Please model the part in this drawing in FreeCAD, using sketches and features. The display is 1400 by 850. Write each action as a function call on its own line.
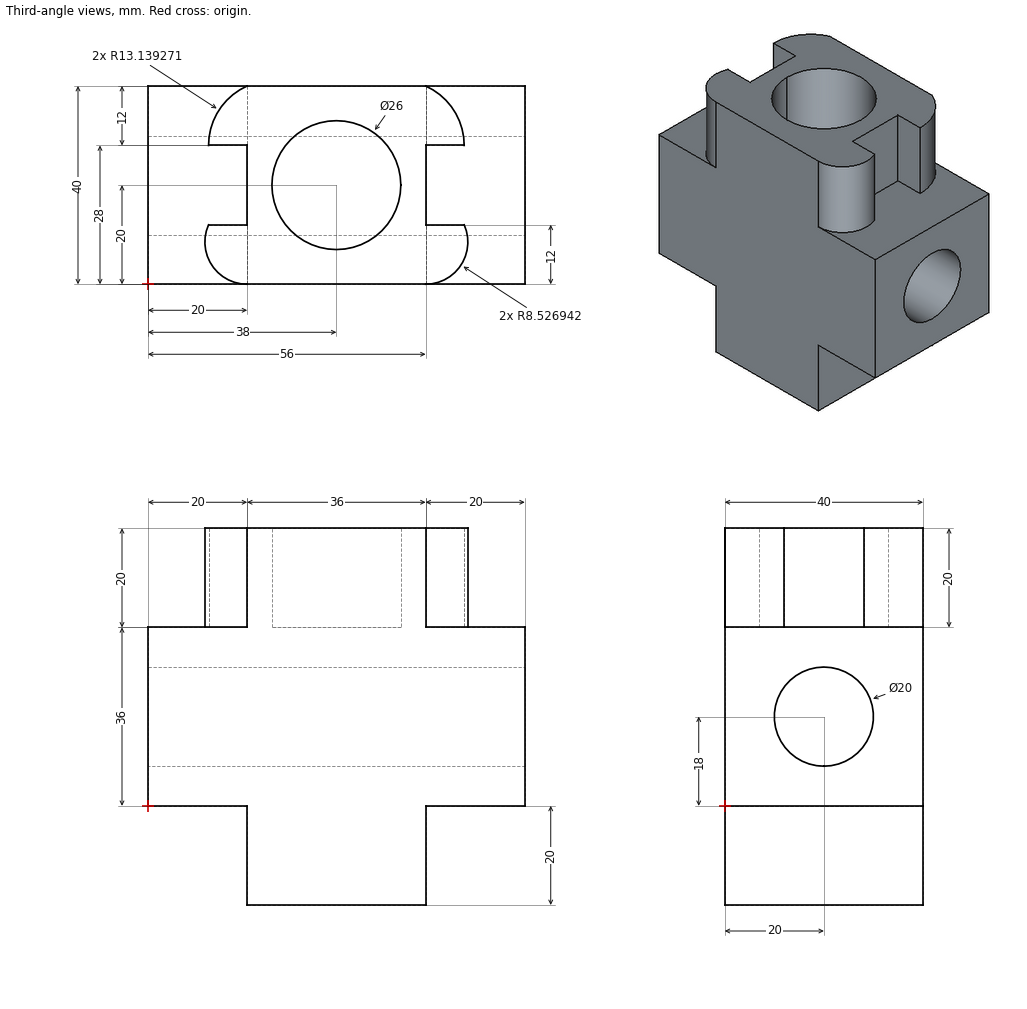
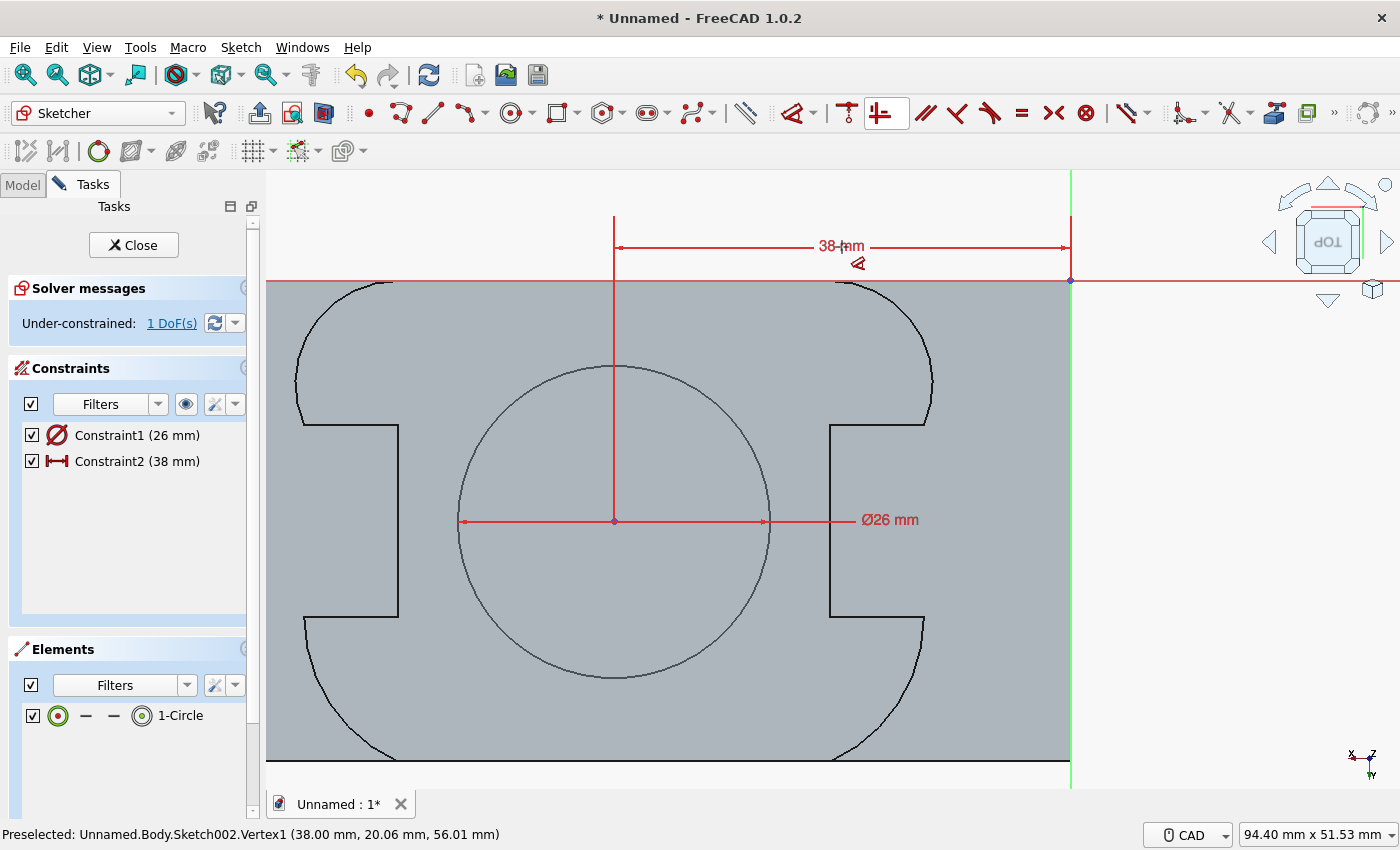
click(614, 522)
click(1105, 401)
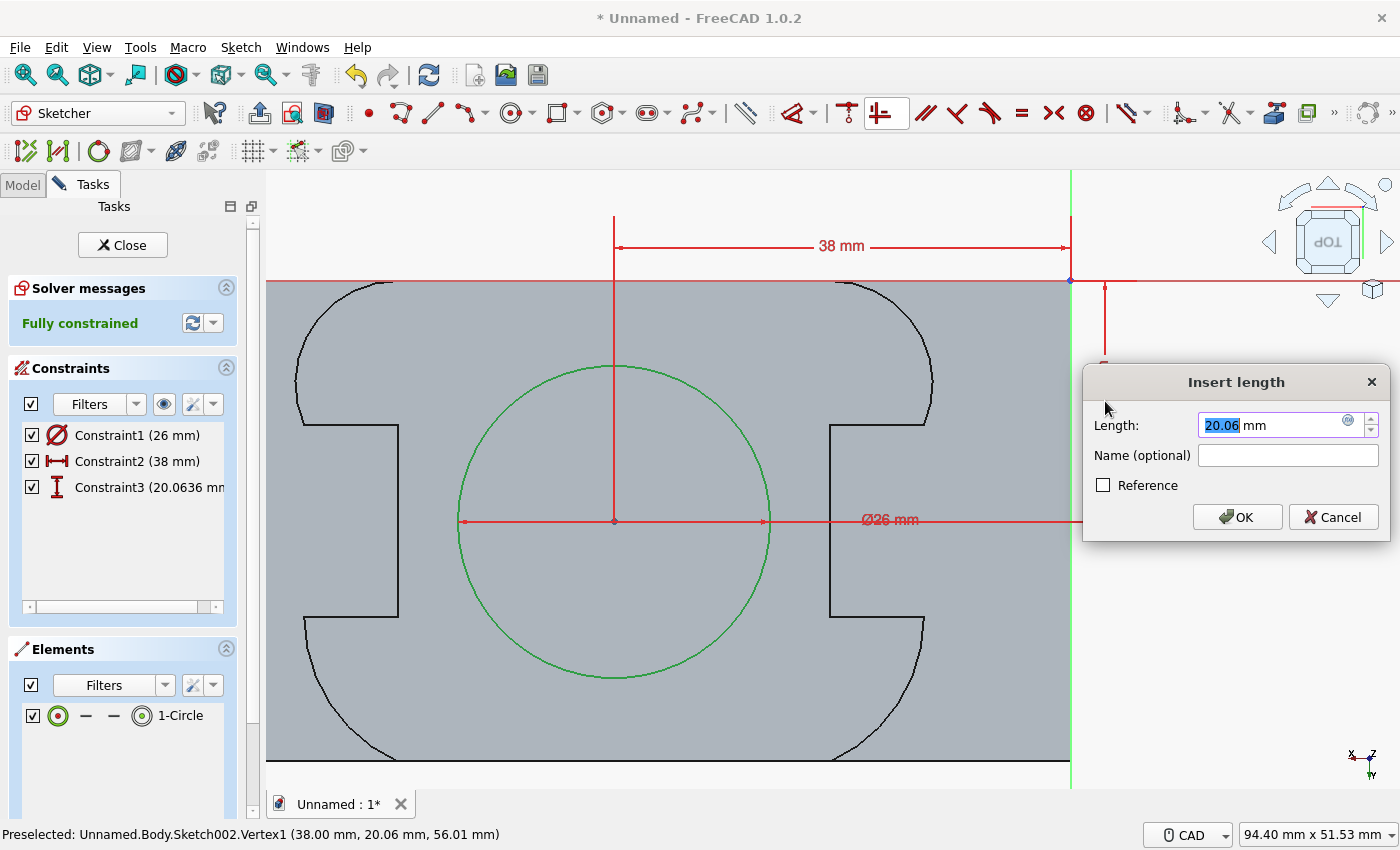
text(20)
key(Return)
key(Escape)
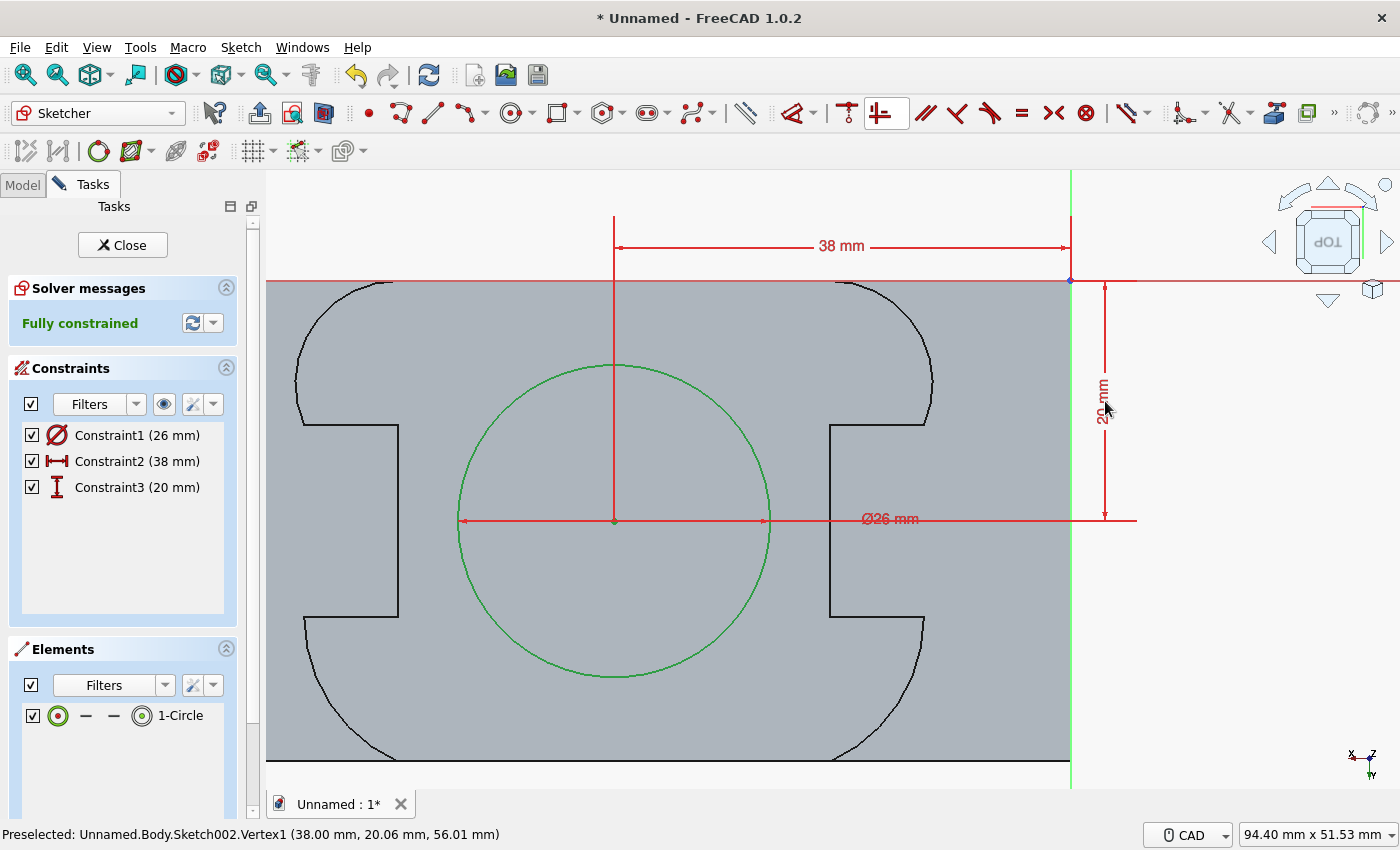
click(123, 245)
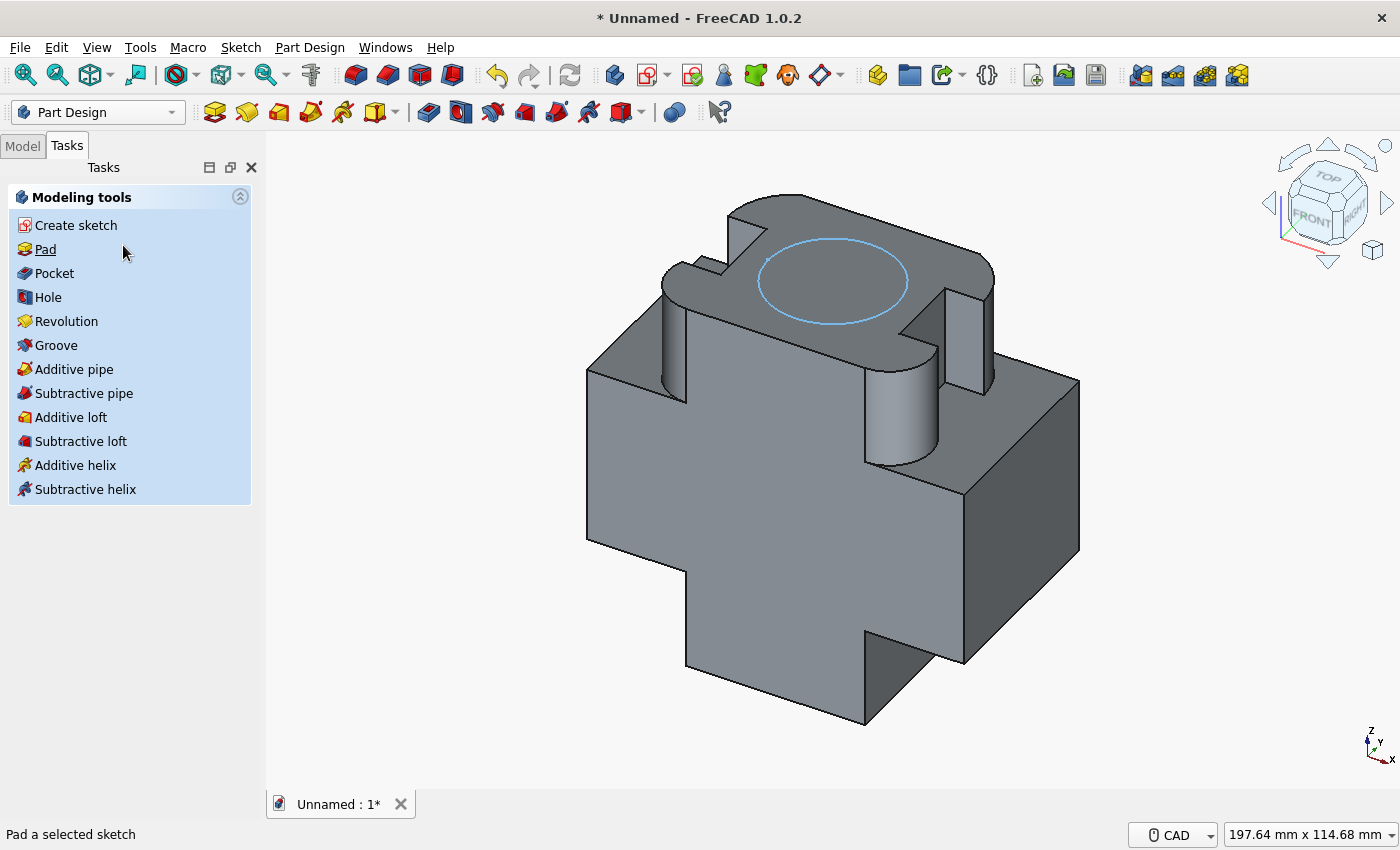
click(430, 112)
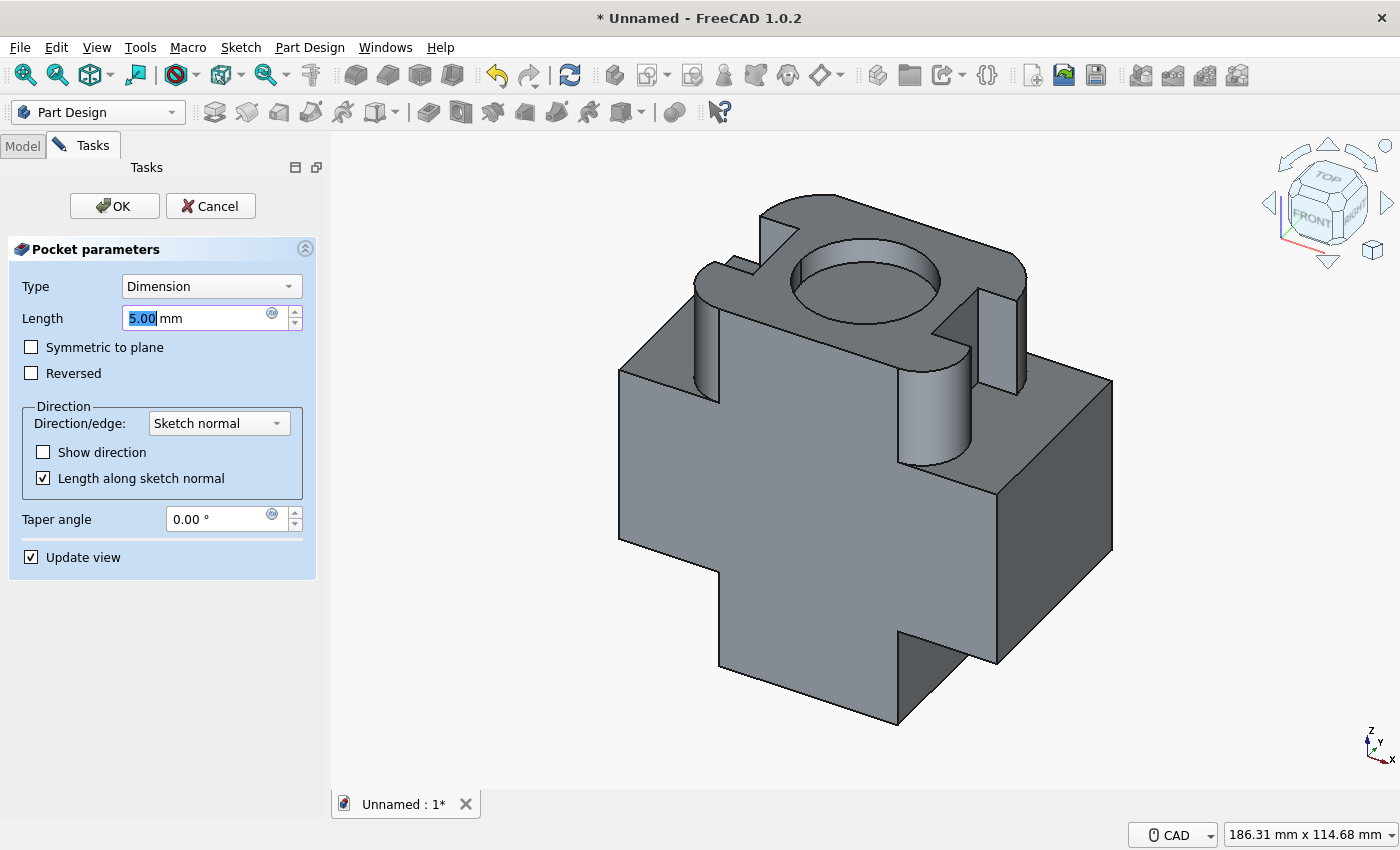
text(20)
key(Tab)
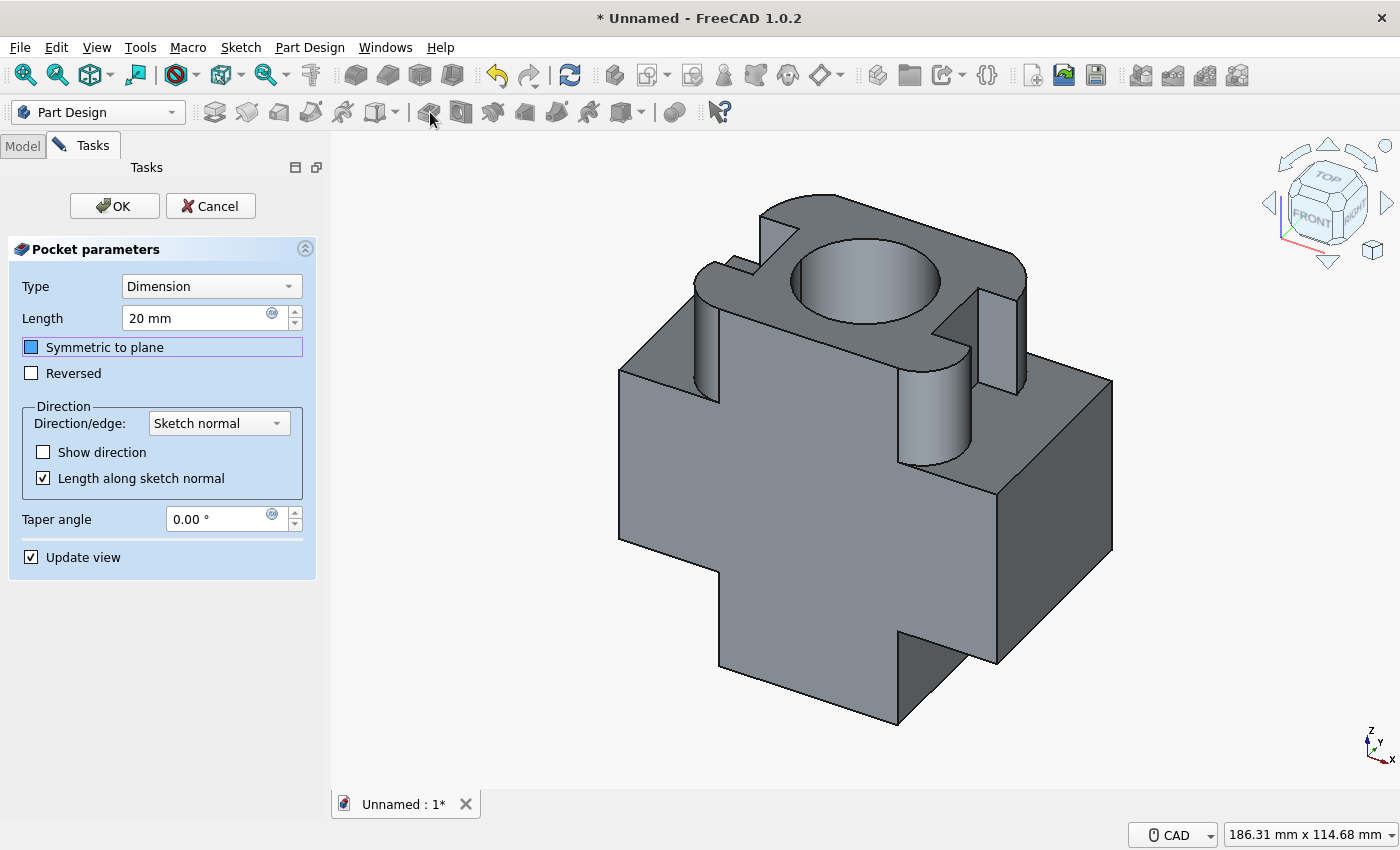
click(115, 206)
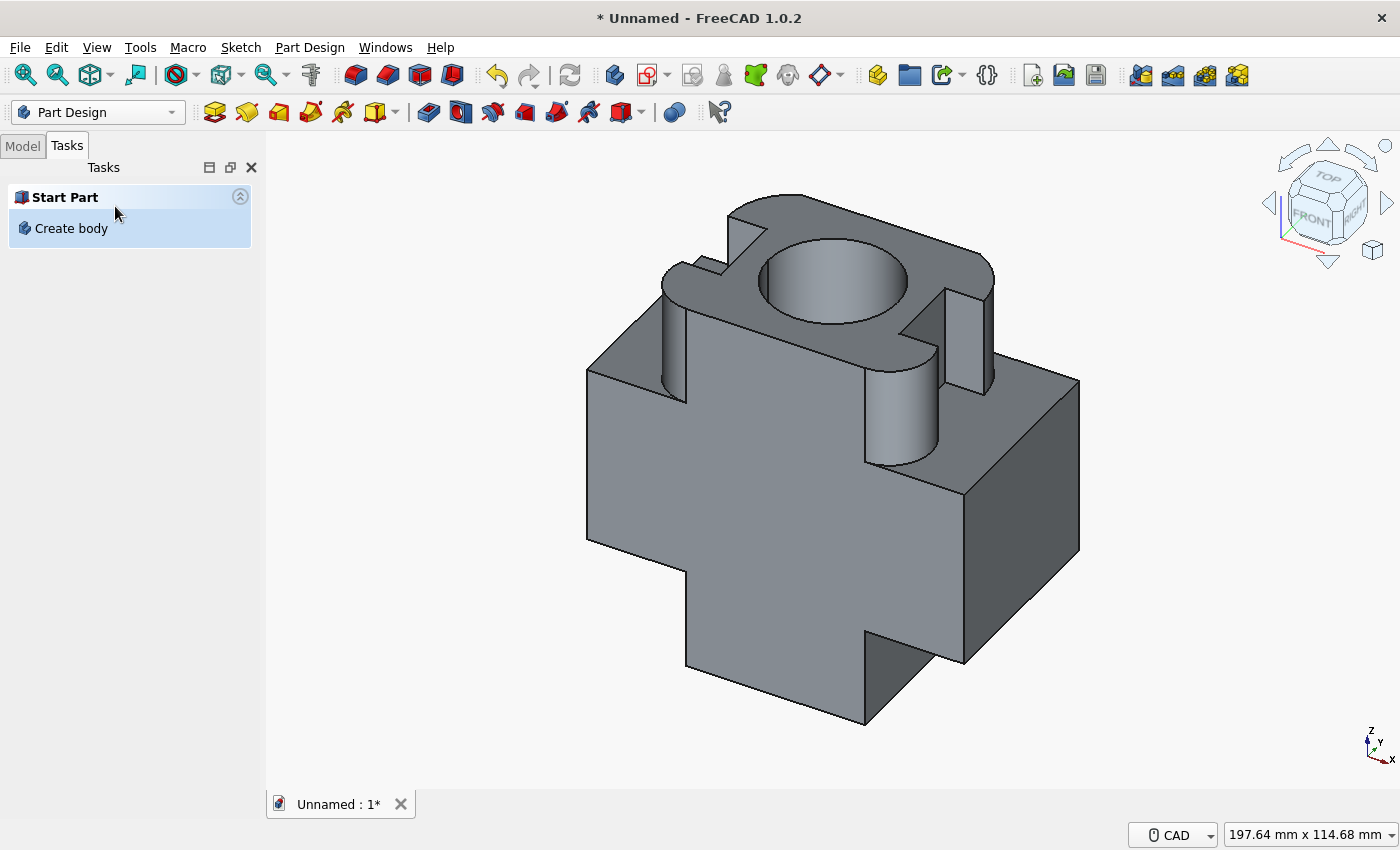
click(1022, 522)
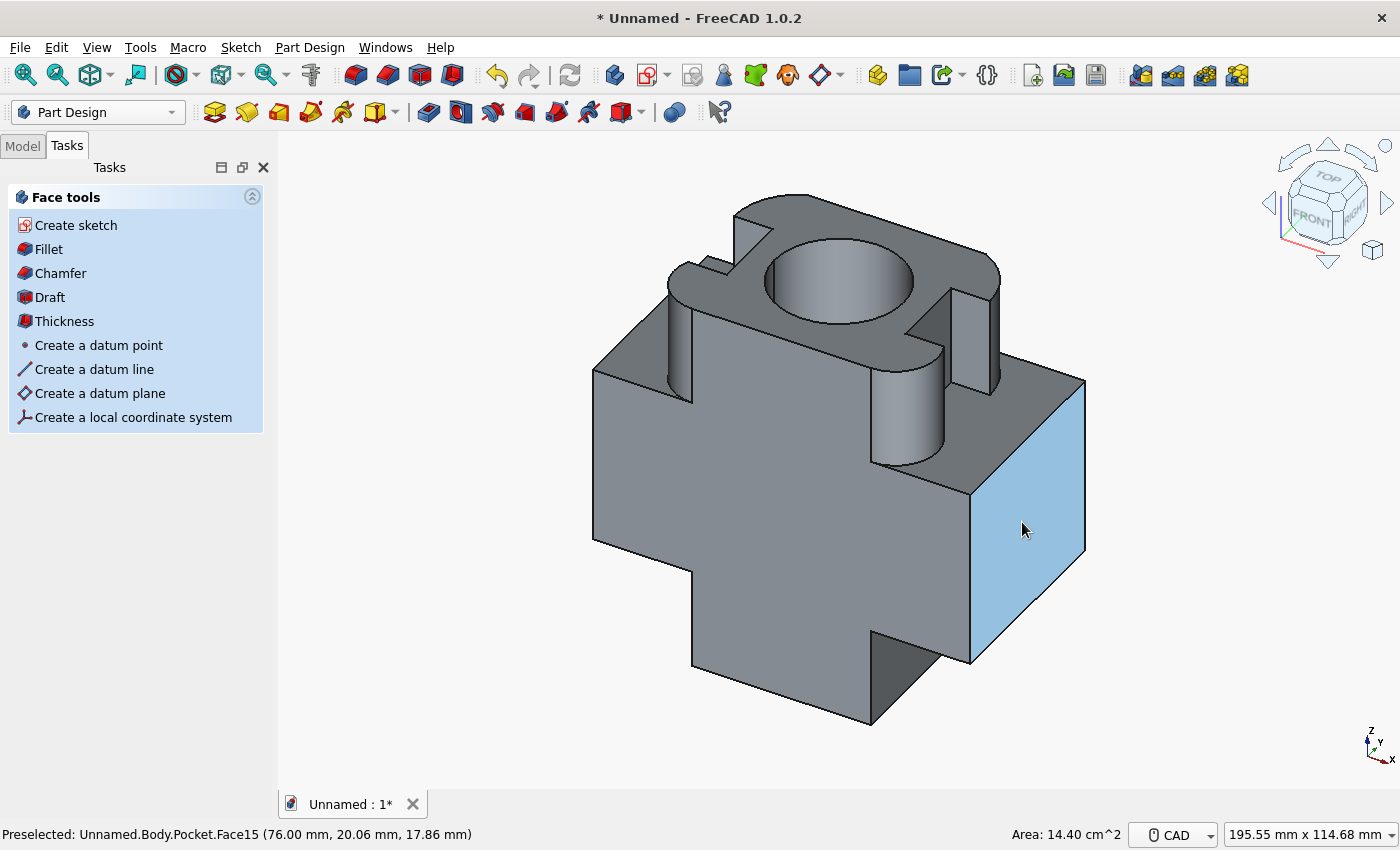
click(648, 76)